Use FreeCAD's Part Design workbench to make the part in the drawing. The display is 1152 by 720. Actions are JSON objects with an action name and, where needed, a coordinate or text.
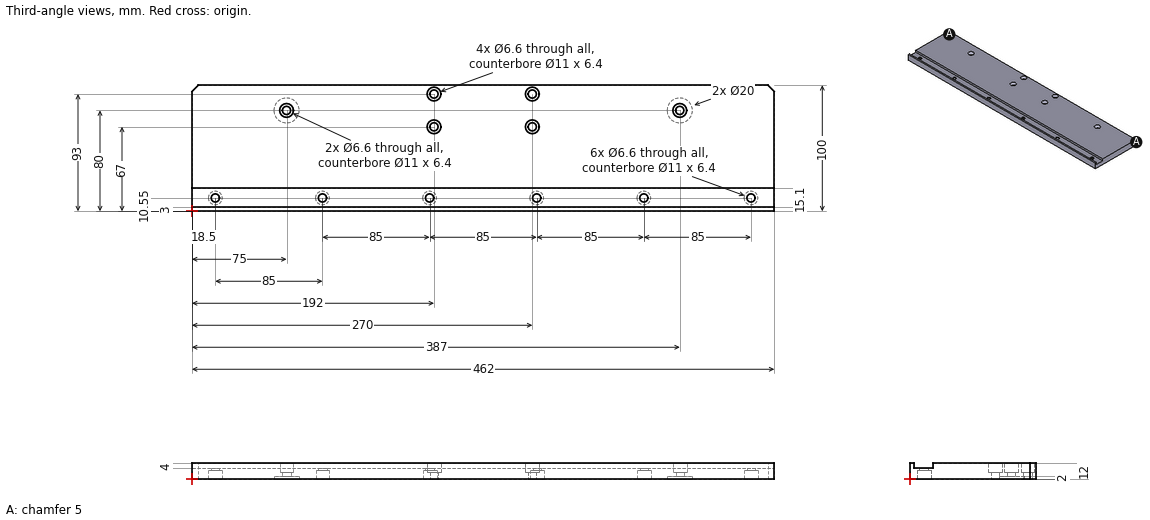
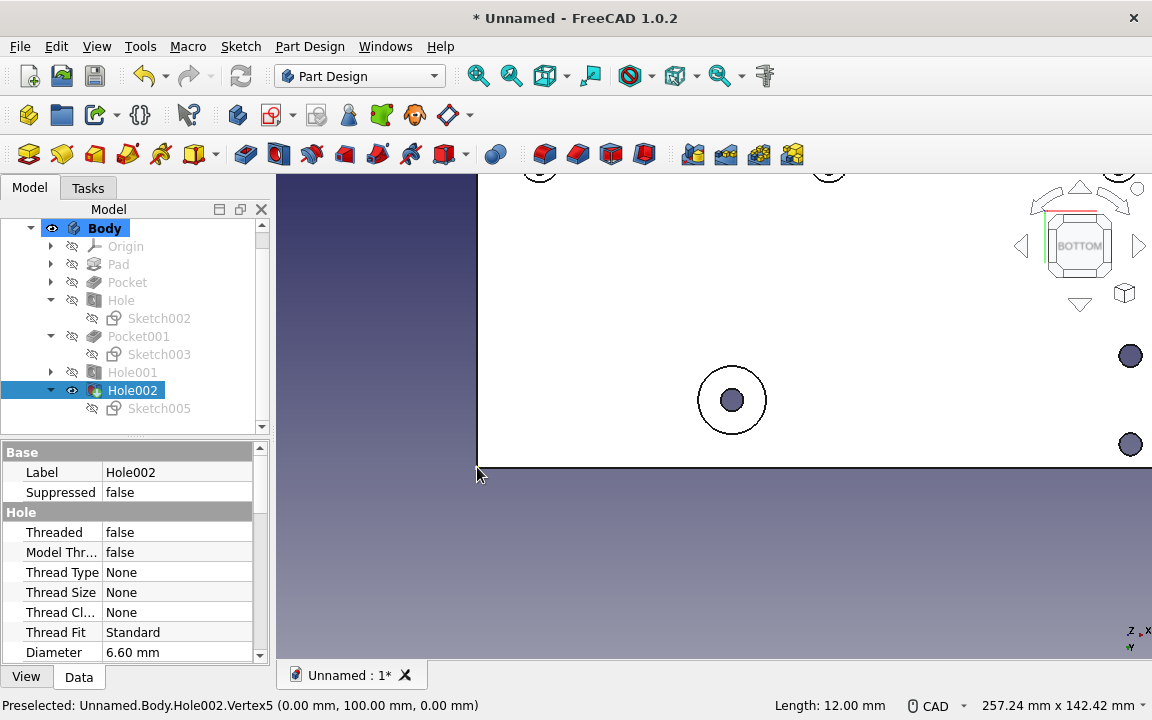
{"action": "key", "text": "v f"}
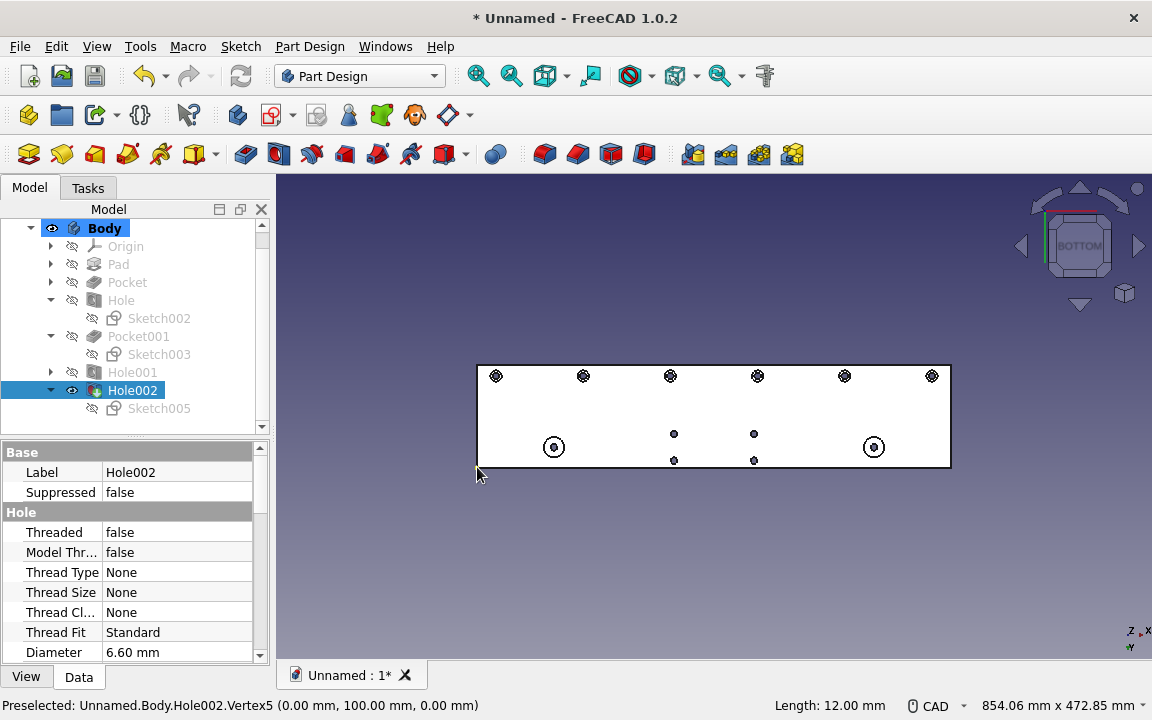
{"action": "key", "text": "4"}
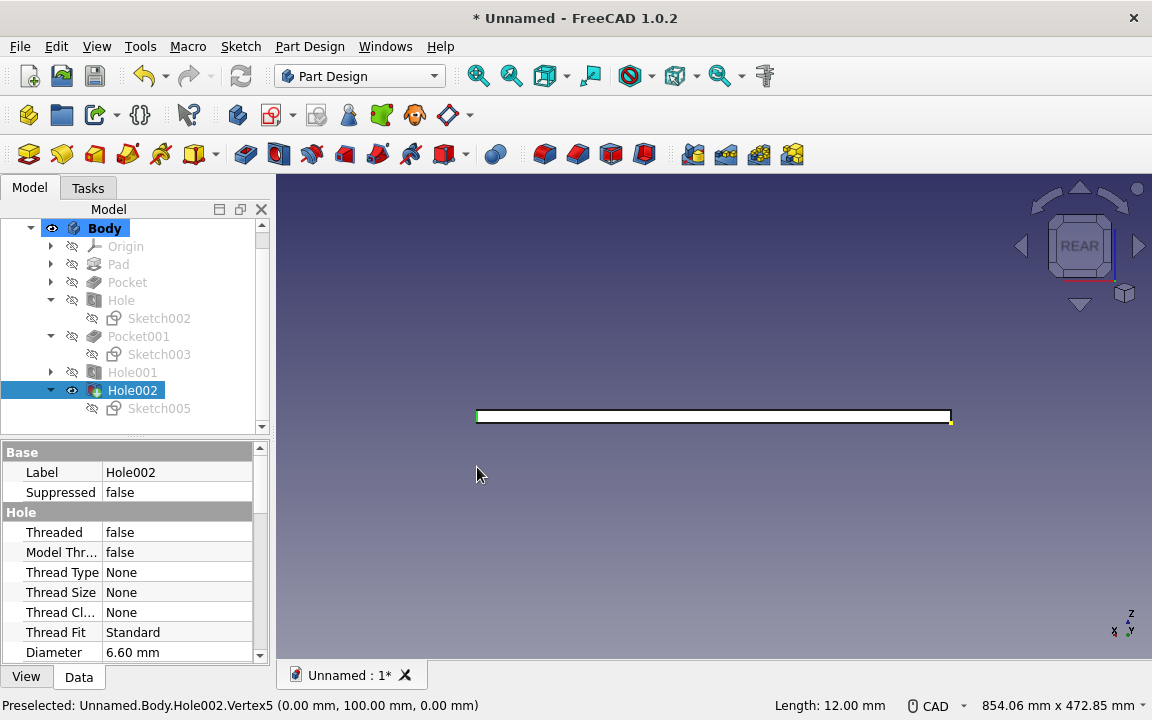
{"action": "scroll", "coordinate": [951, 416], "scroll_direction": "up", "scroll_amount": 6}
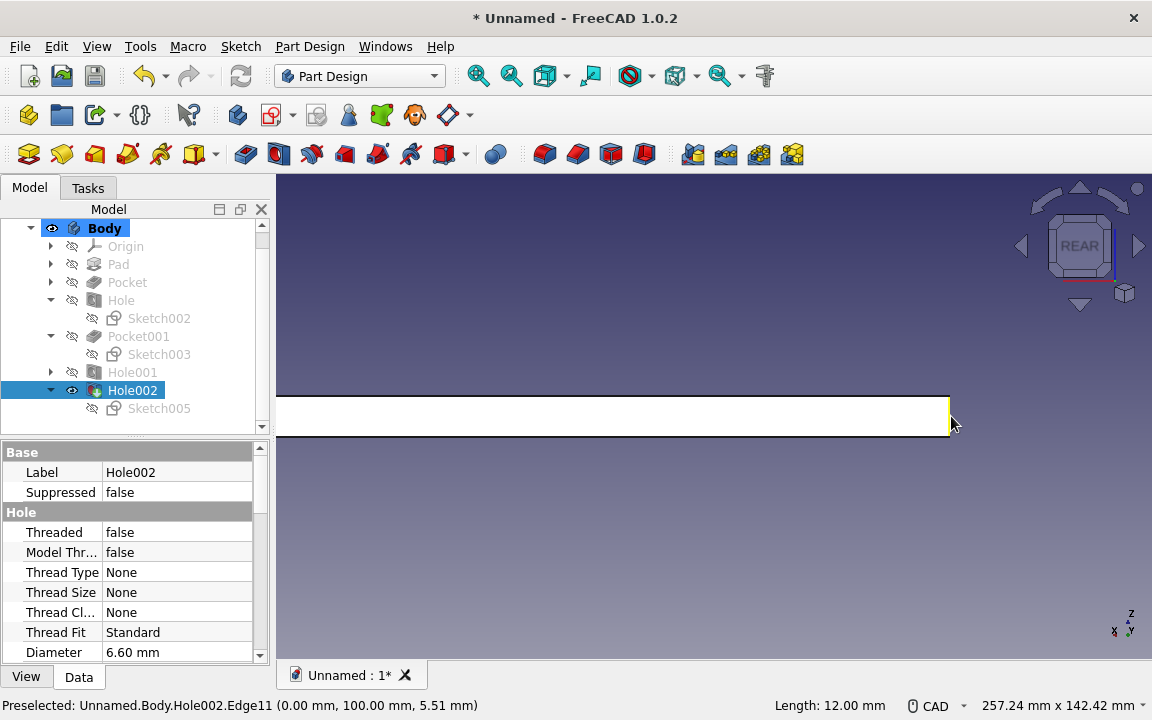
{"action": "left_click", "coordinate": [949, 416], "text": "ctrl"}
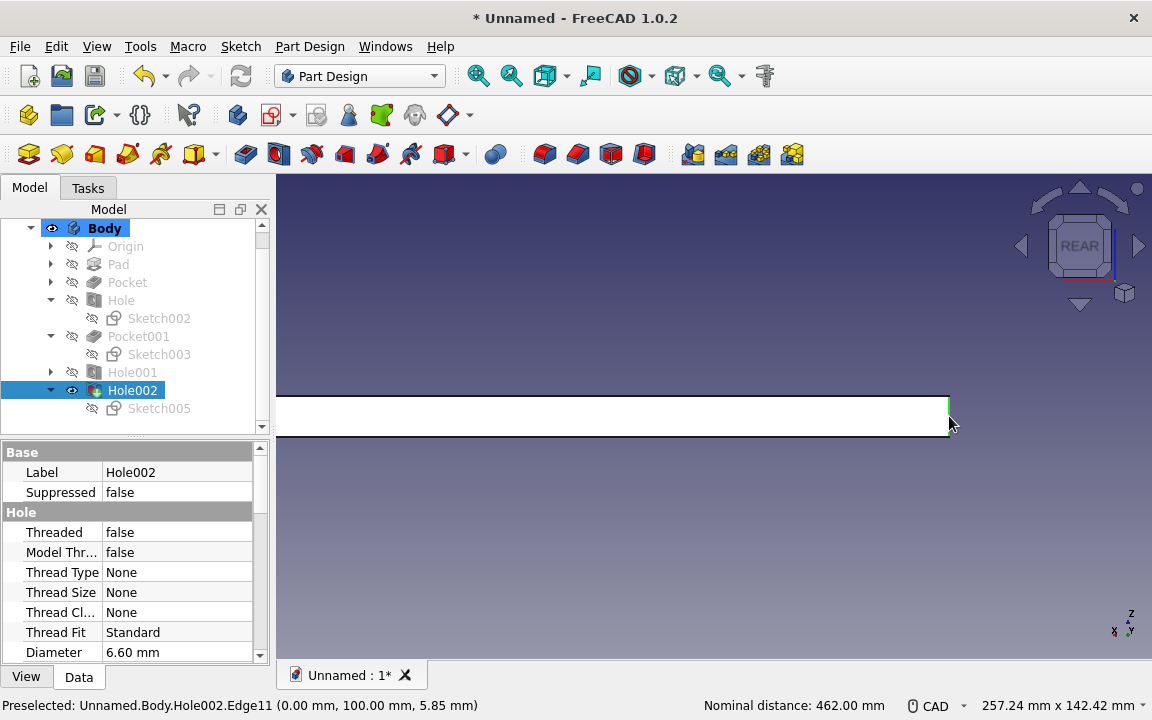
{"action": "left_click", "coordinate": [578, 154]}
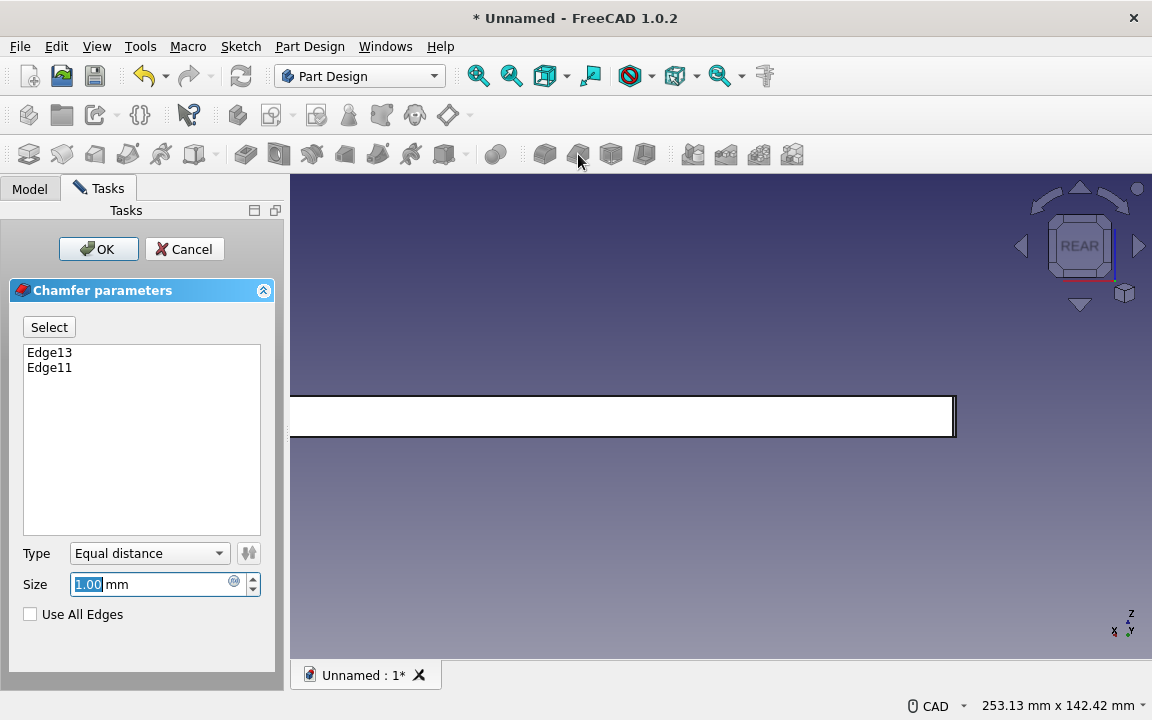
{"action": "type", "text": "5"}
{"action": "key", "text": "Tab"}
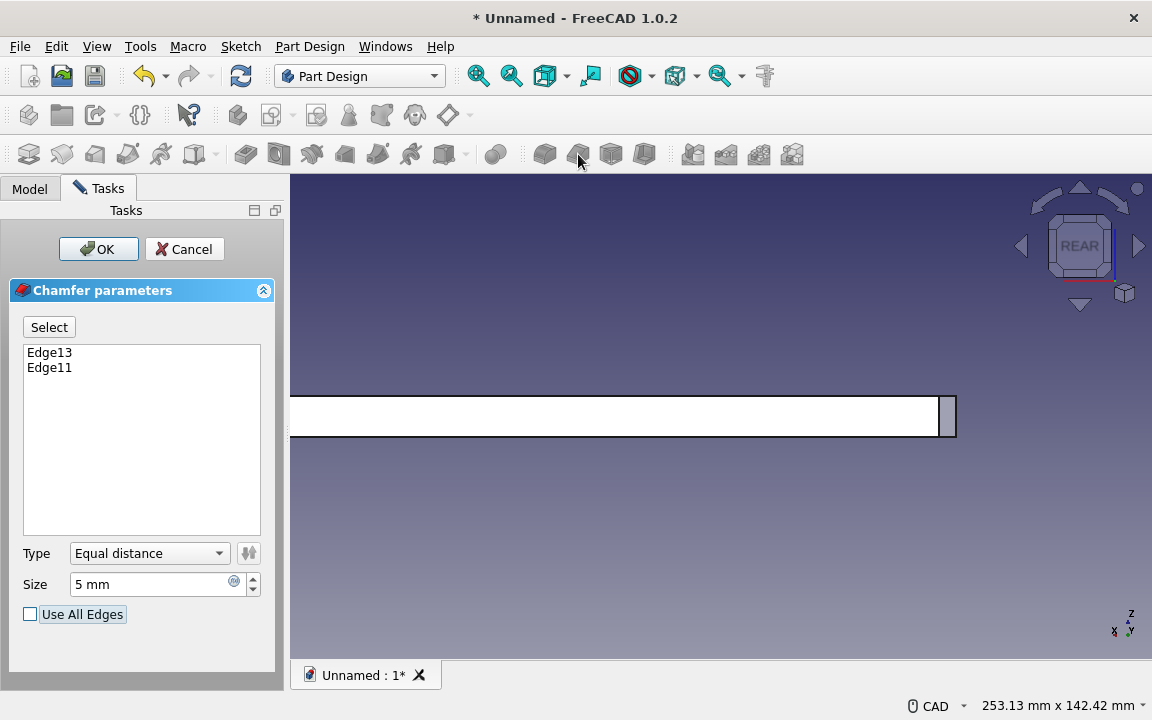
{"action": "left_click", "coordinate": [99, 249]}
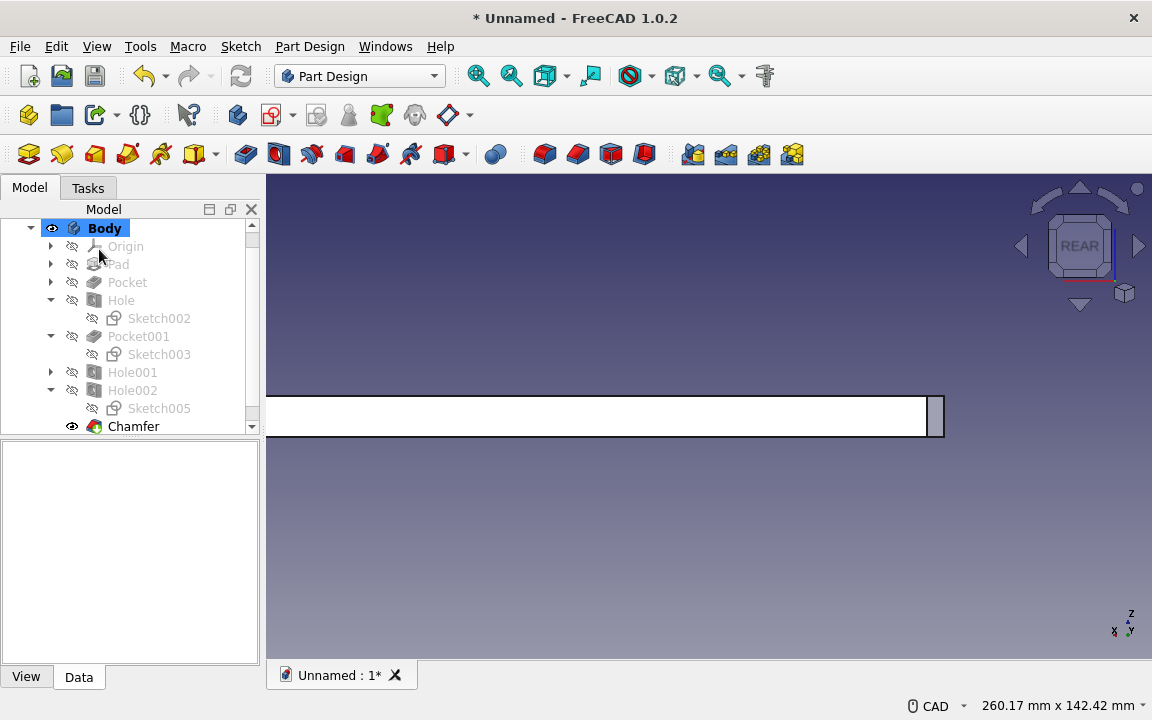
{"action": "key", "text": "0"}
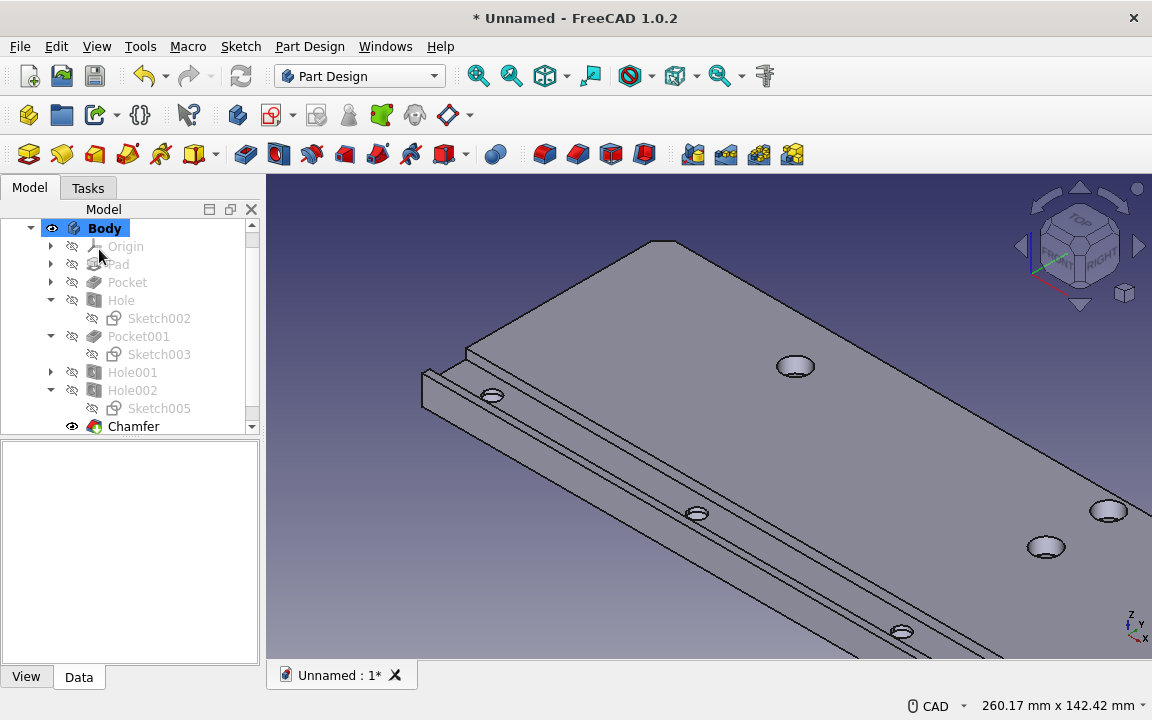
{"action": "left_click", "coordinate": [479, 76]}